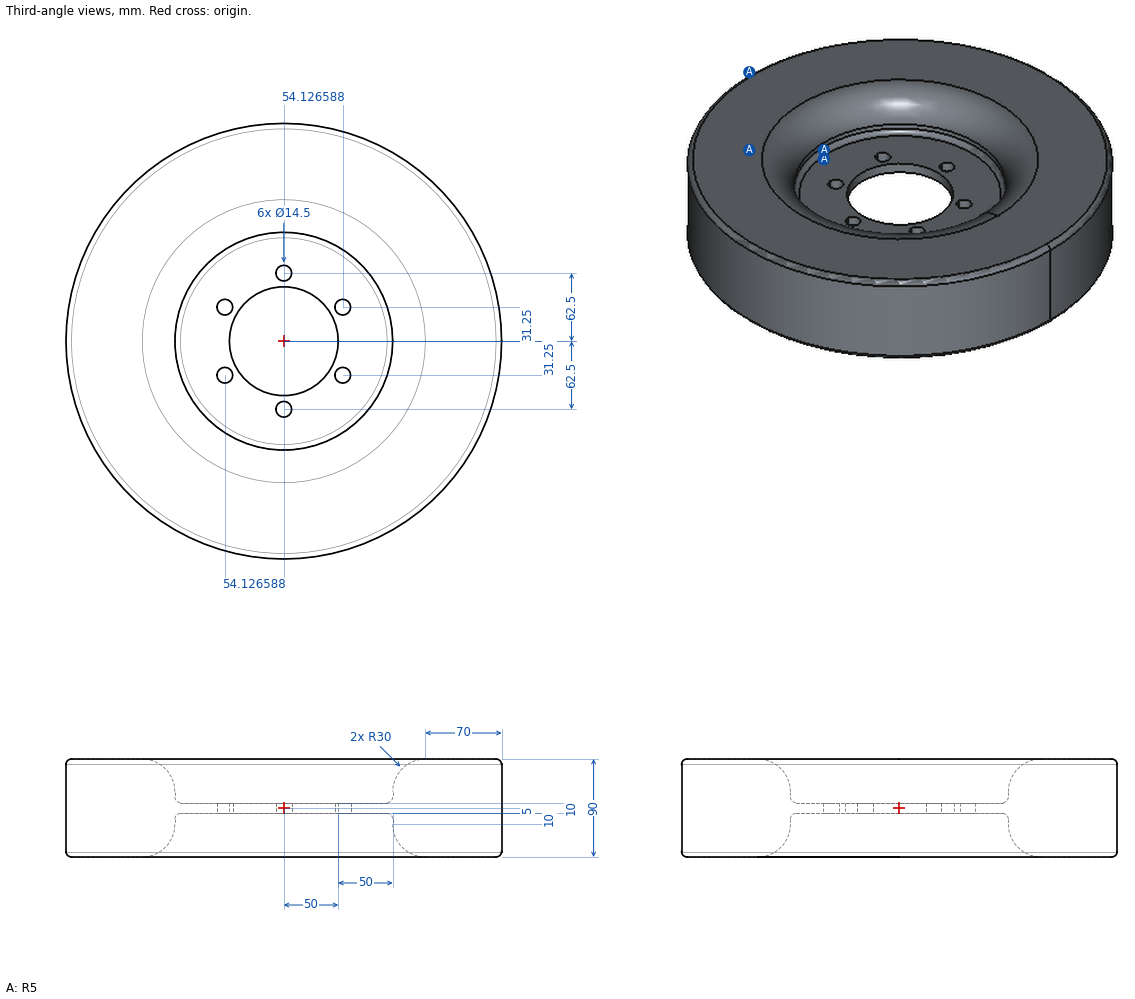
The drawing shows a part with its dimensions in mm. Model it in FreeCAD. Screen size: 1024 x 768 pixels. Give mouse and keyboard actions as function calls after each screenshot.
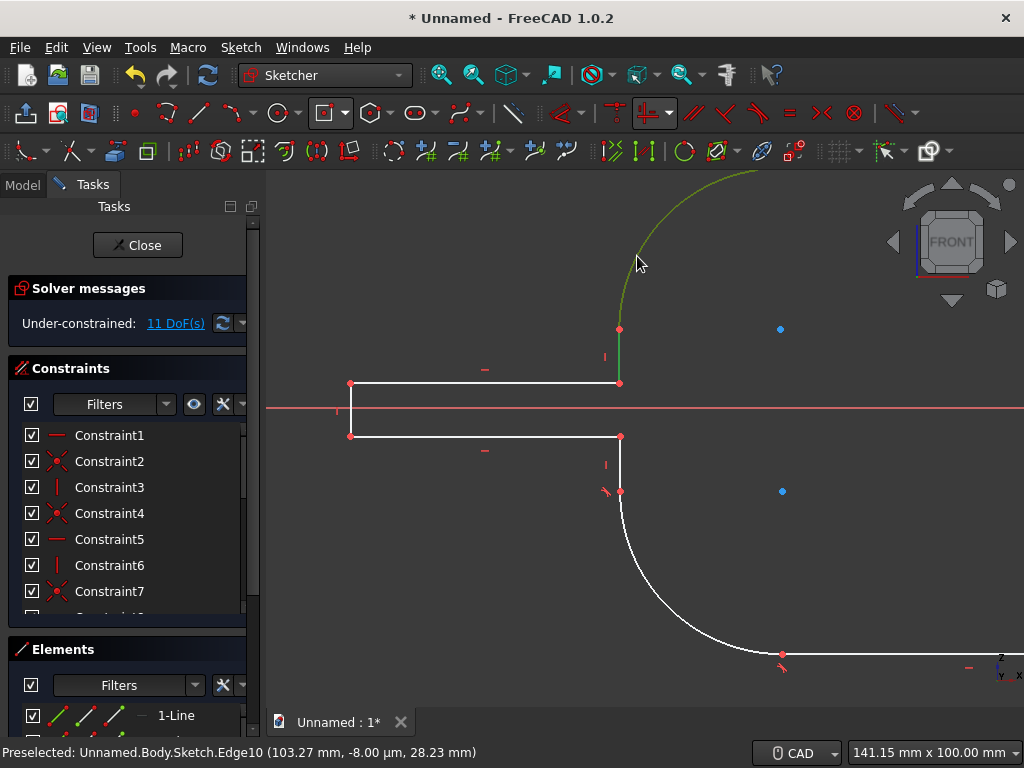
click(758, 114)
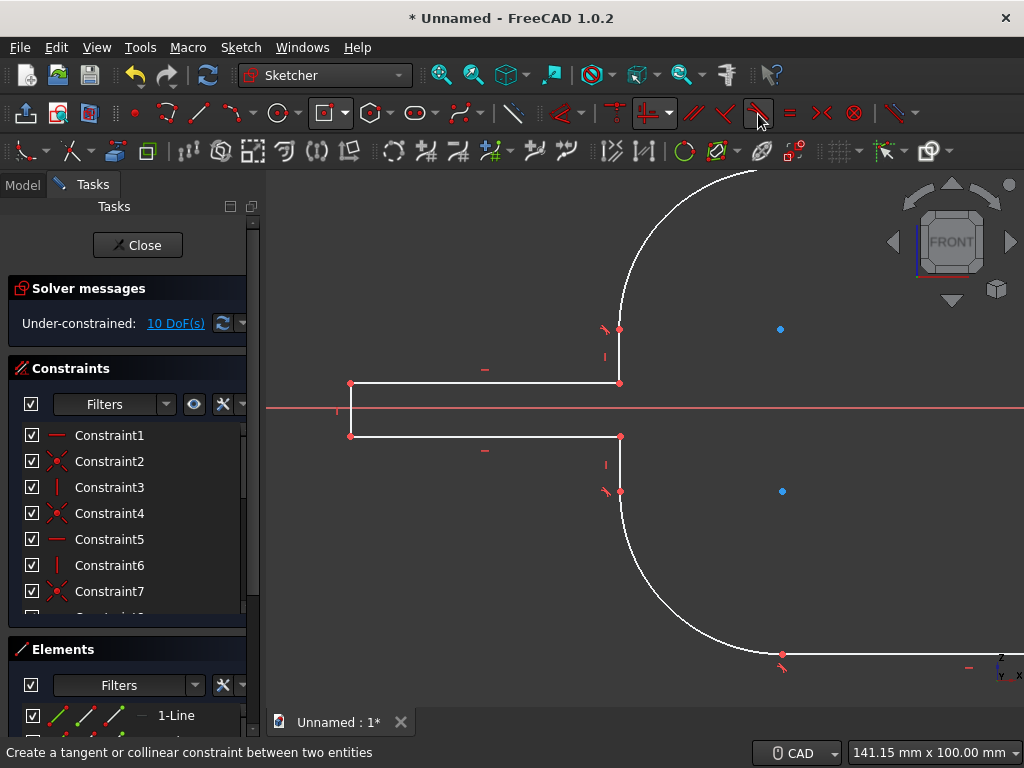
click(638, 566)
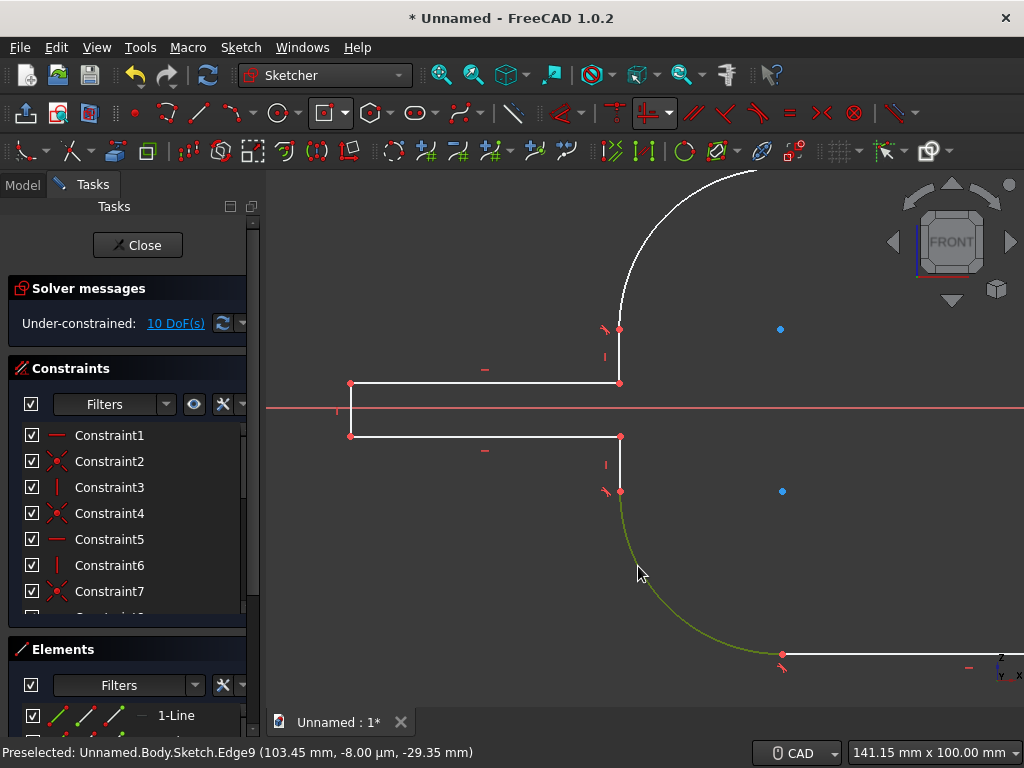
click(637, 256)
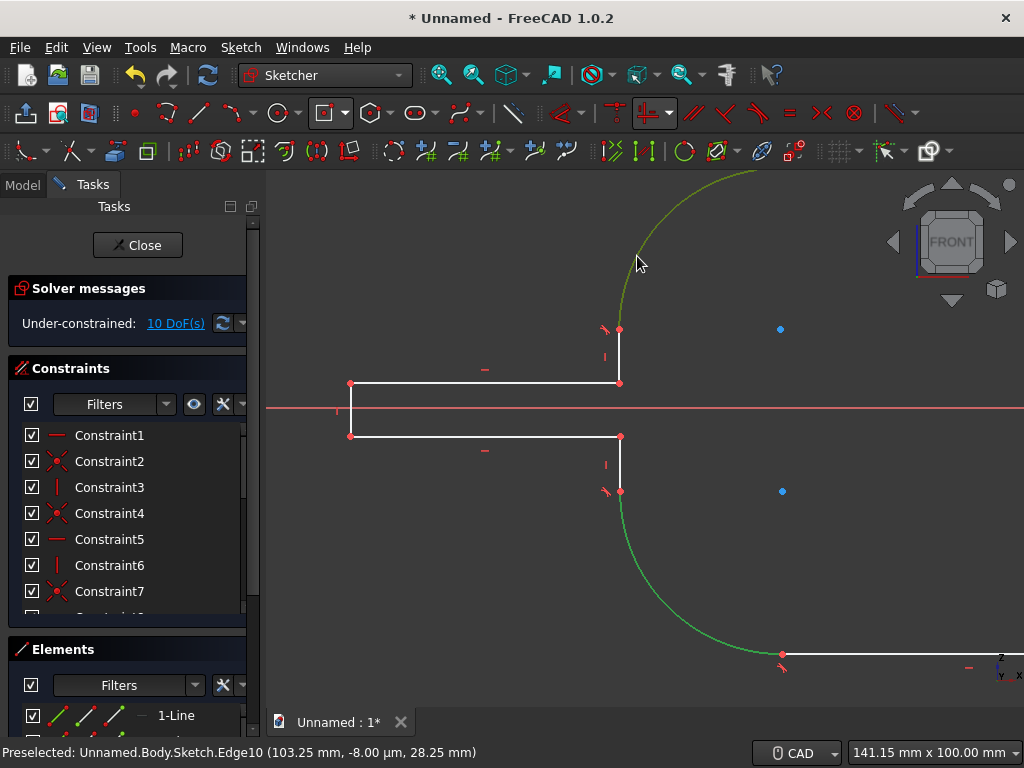
click(790, 114)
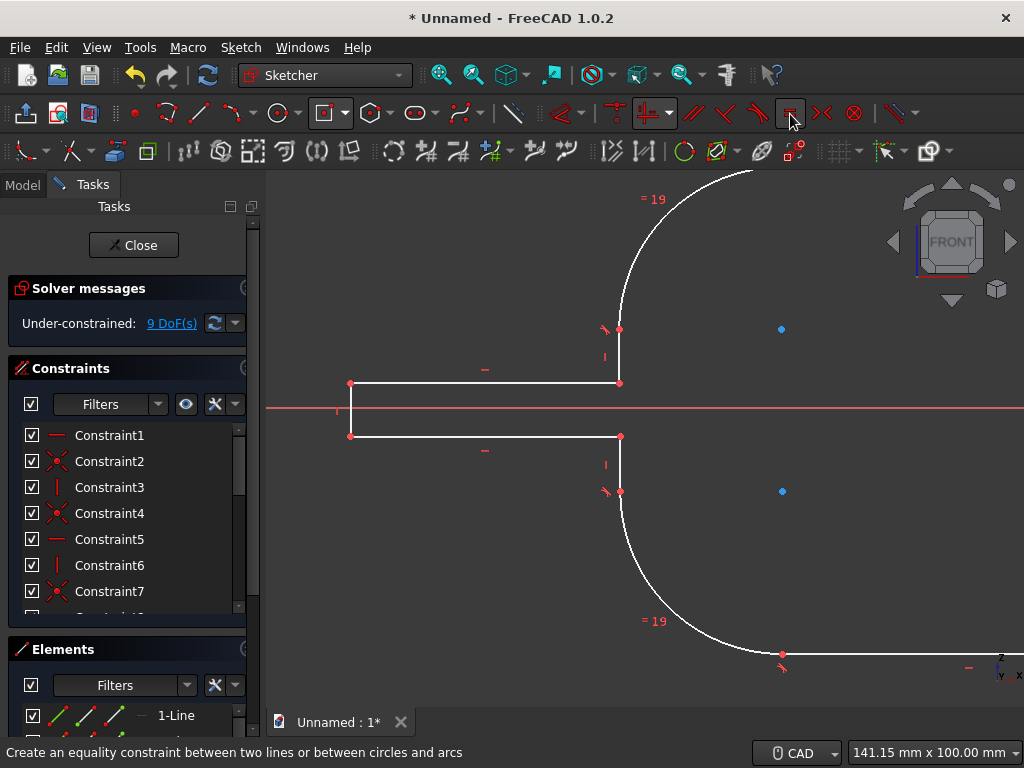
click(638, 565)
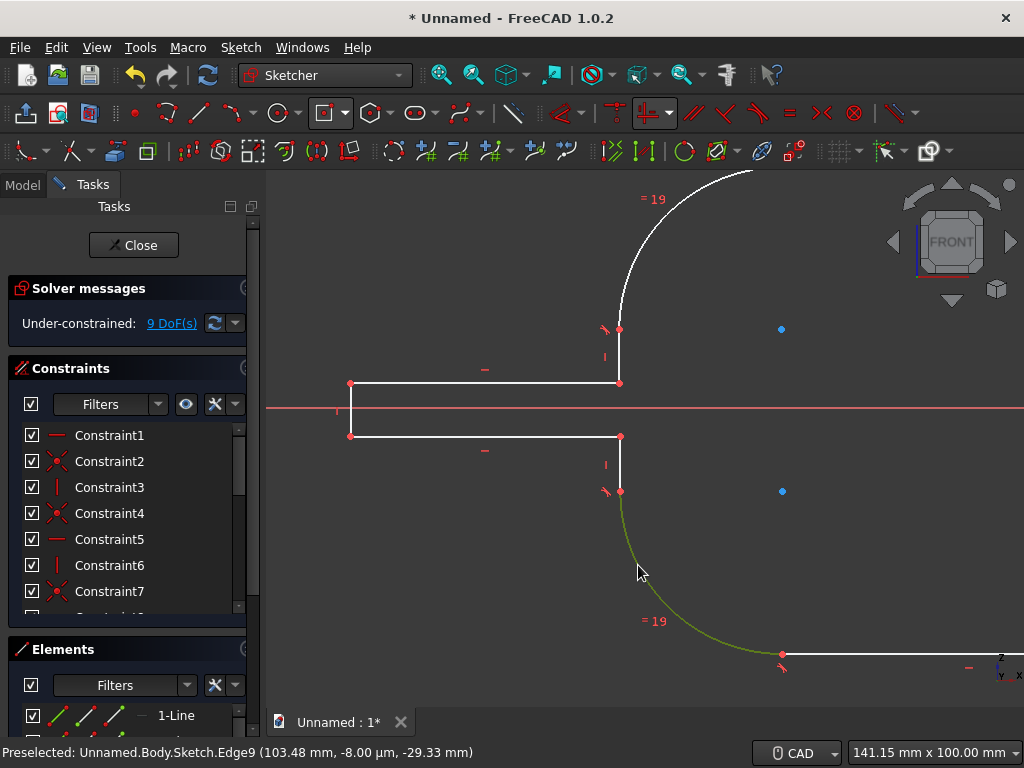
click(584, 114)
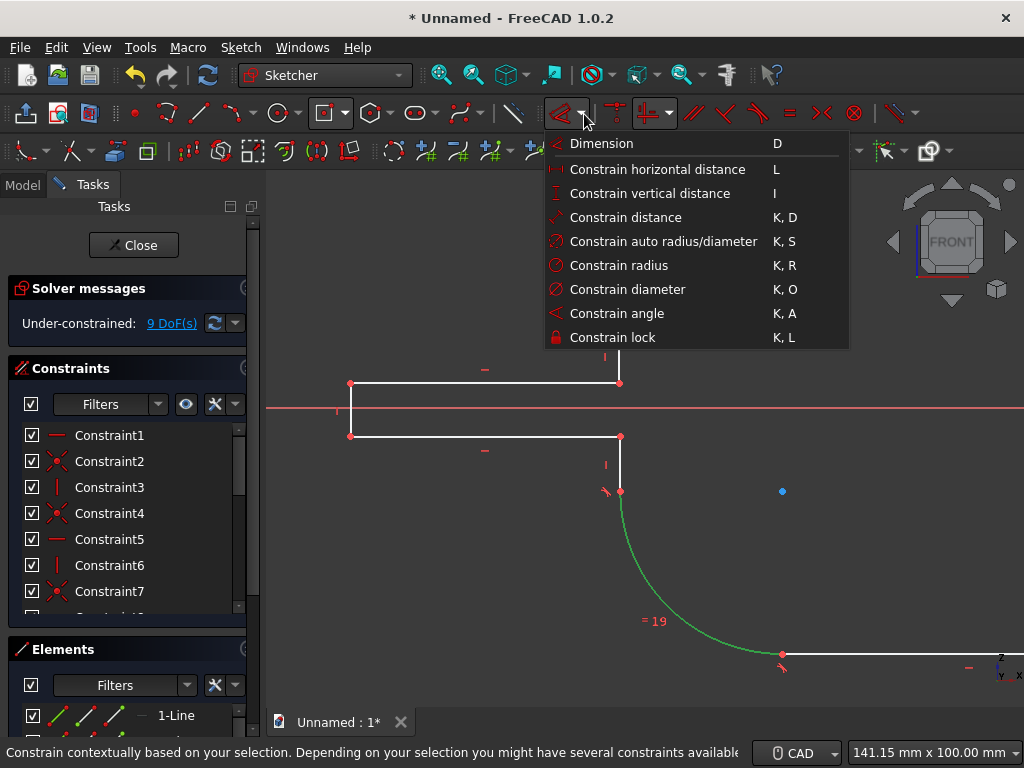
click(697, 265)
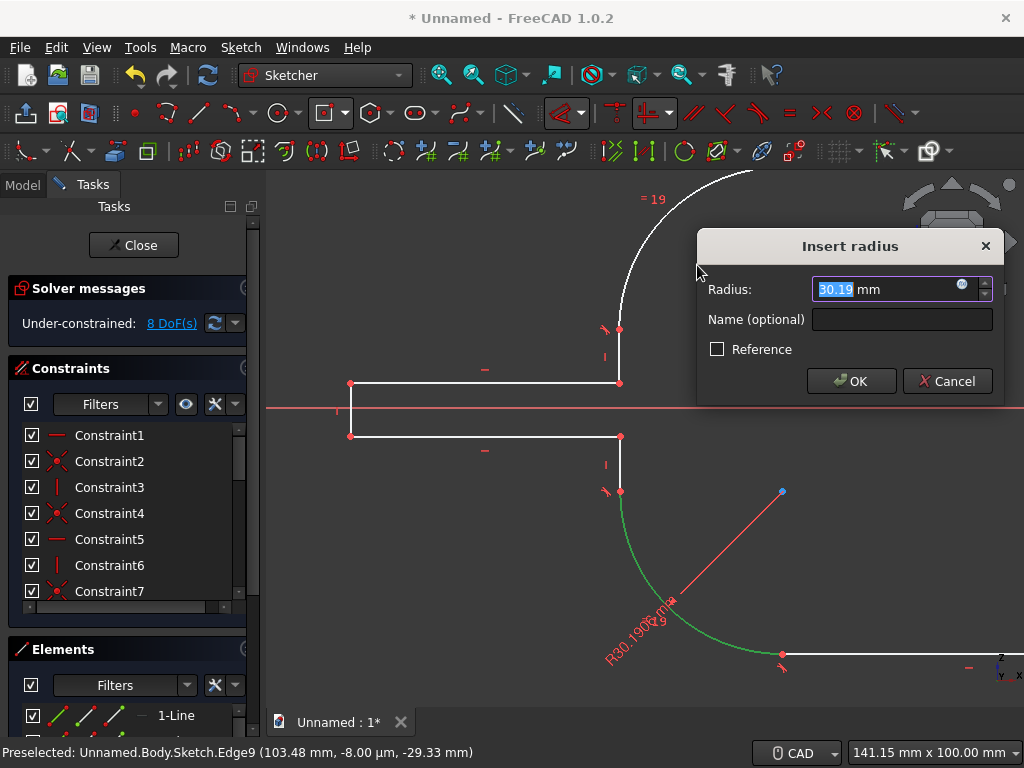
text(30)
key(Return)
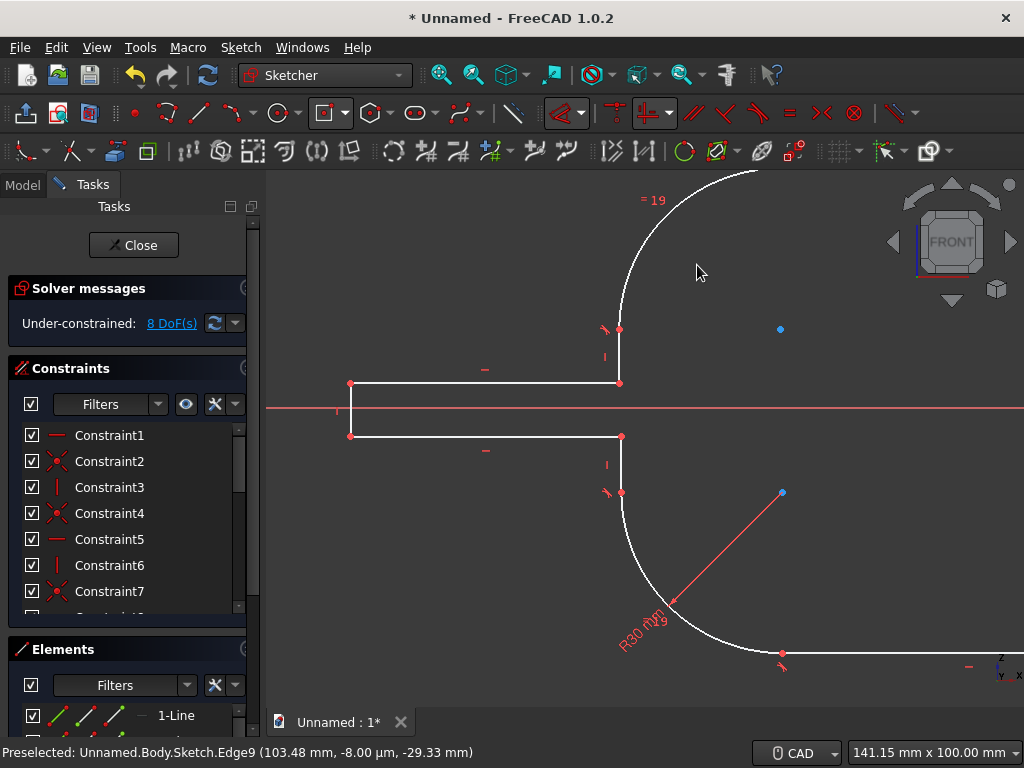
scroll(552, 456, down, 5)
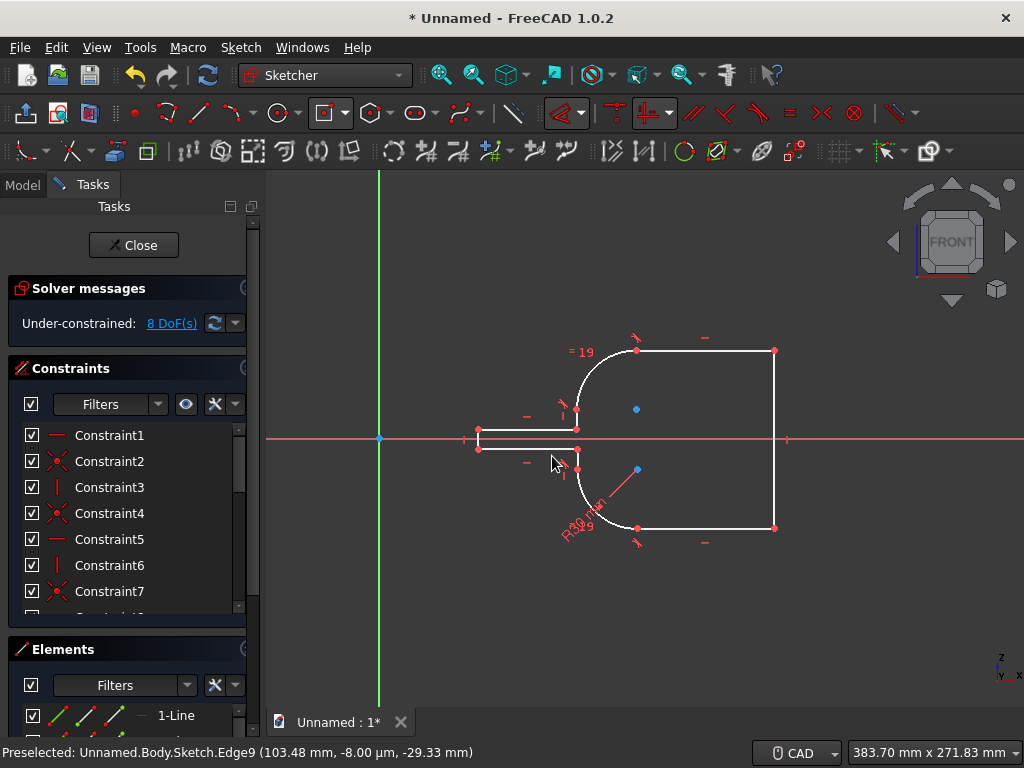
click(678, 351)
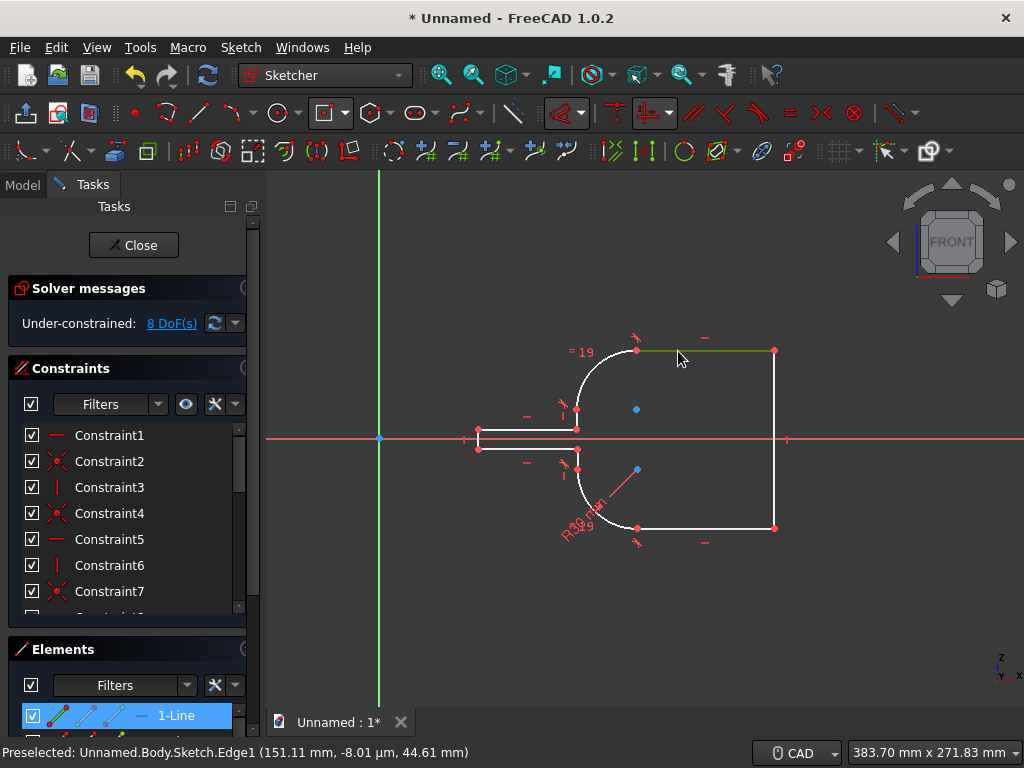
key(l)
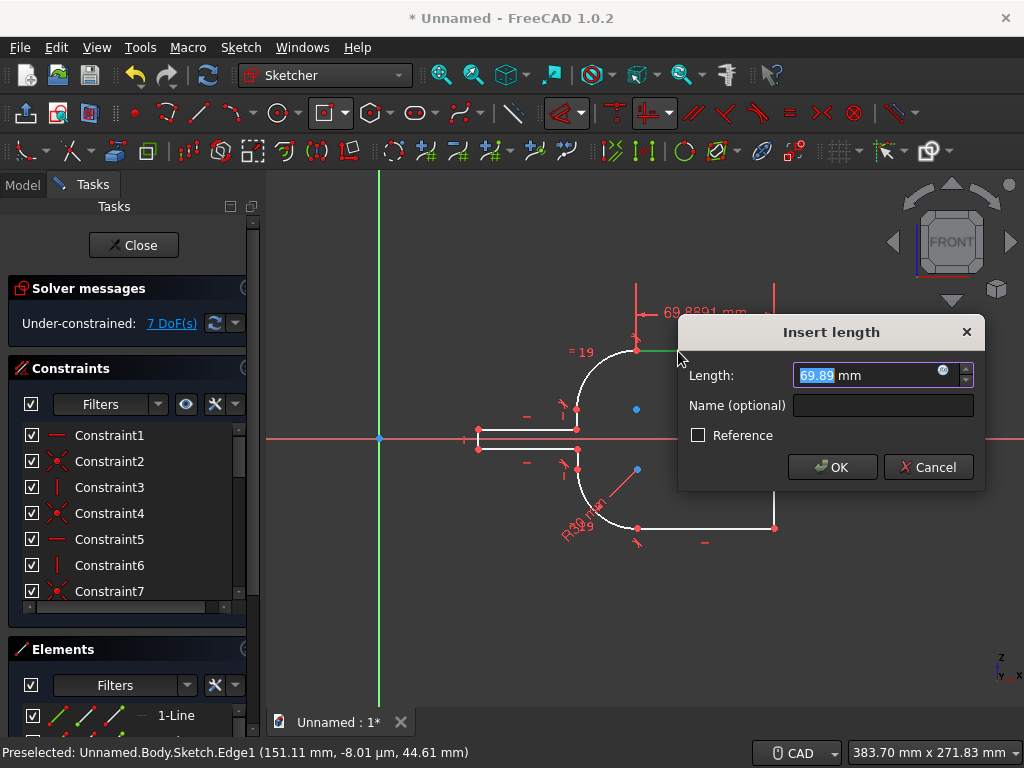
text(70)
key(Return)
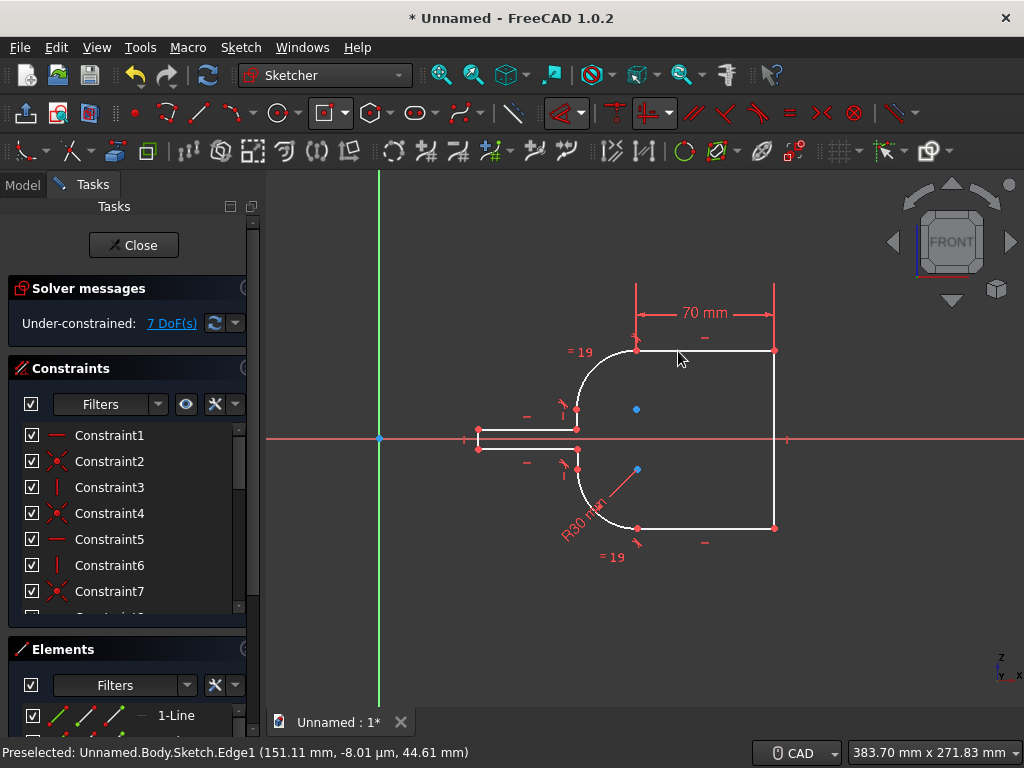
click(774, 404)